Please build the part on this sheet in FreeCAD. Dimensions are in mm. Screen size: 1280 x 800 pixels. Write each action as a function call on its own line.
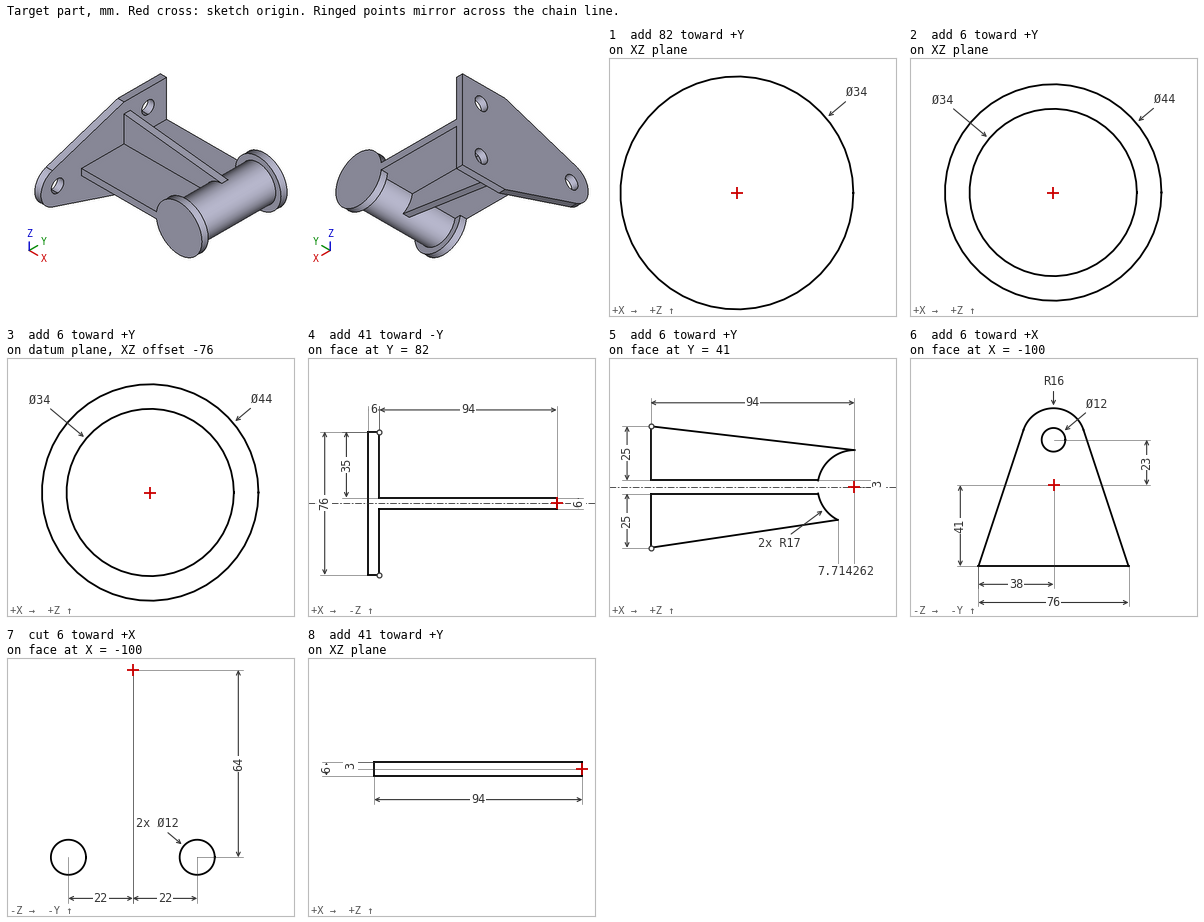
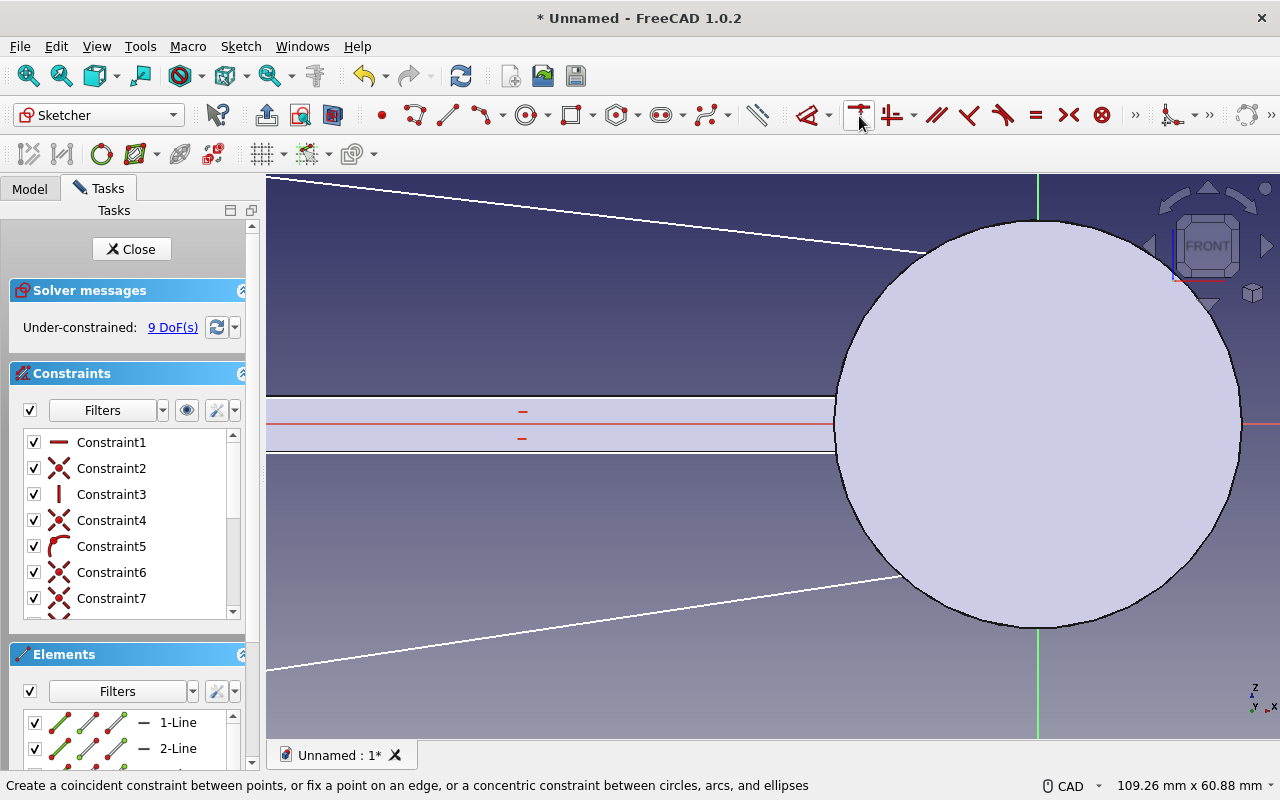
click(973, 280)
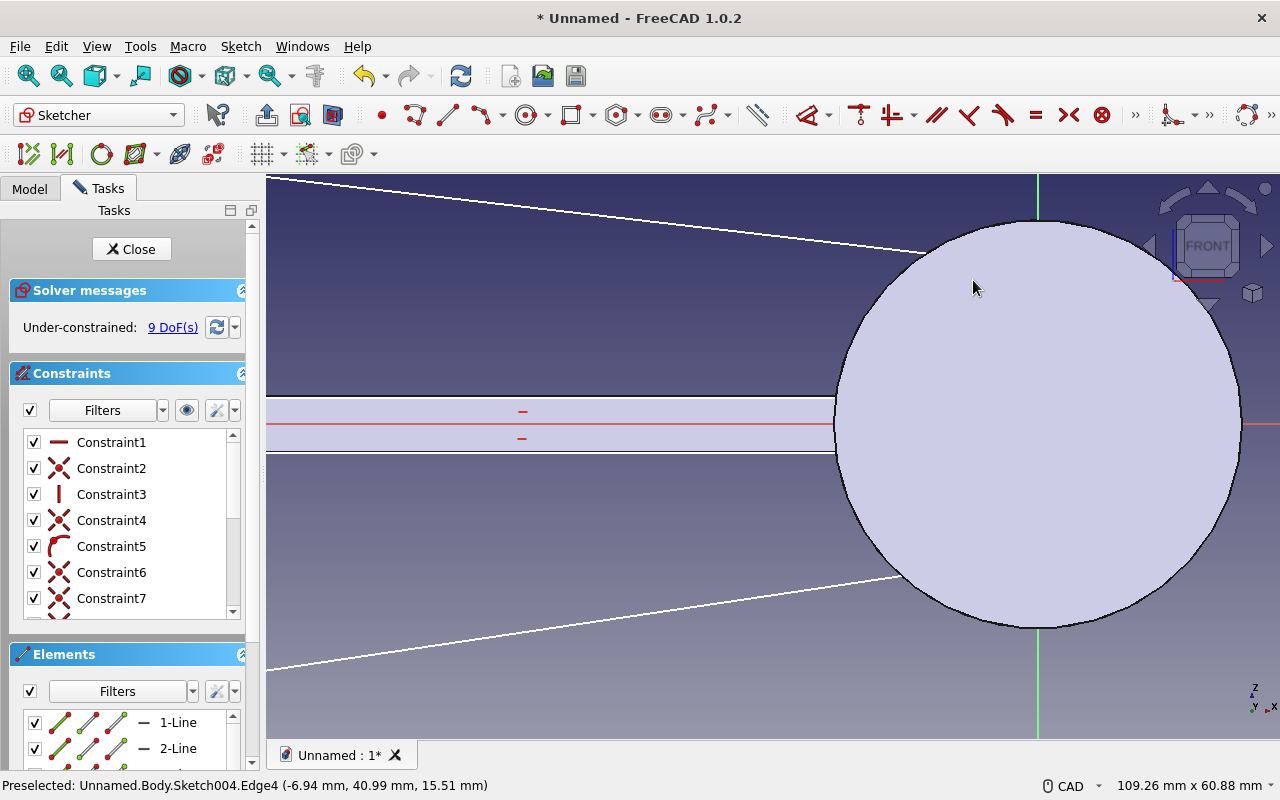
click(895, 495)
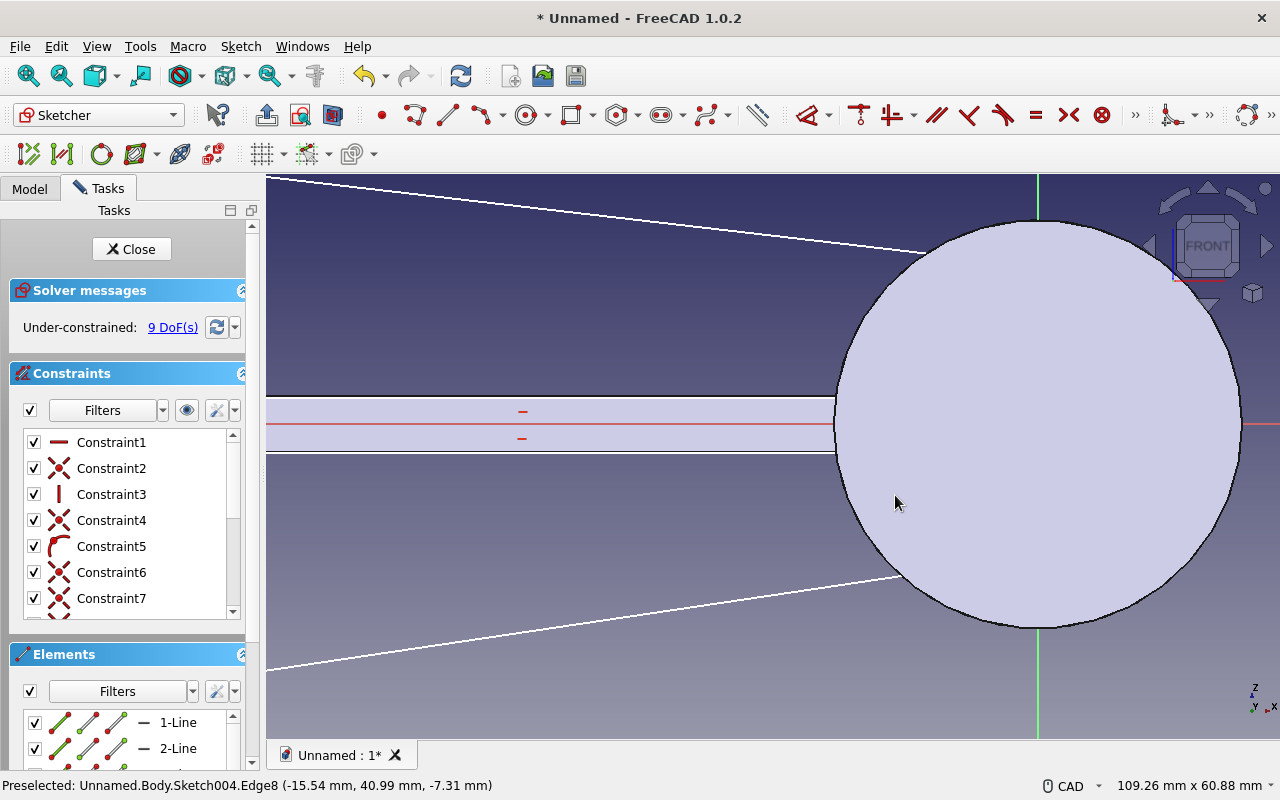
click(1036, 116)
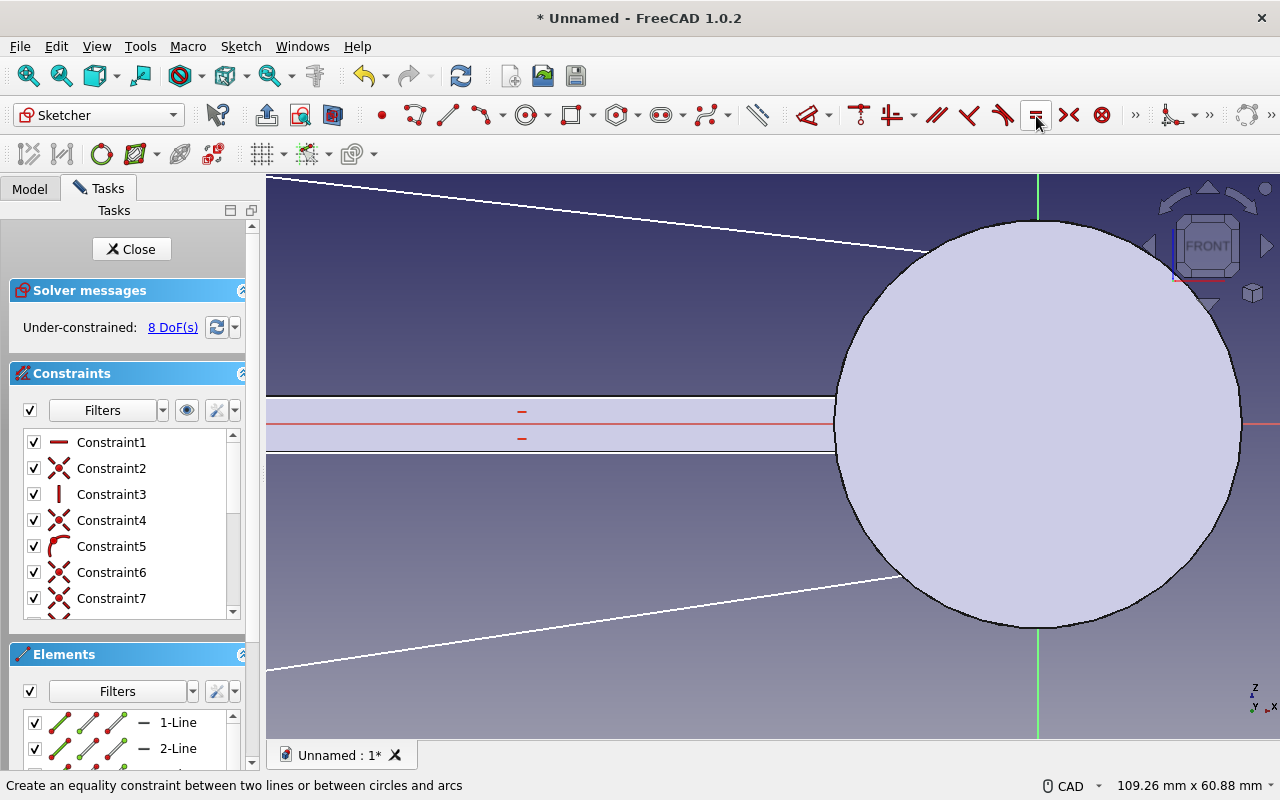
scroll(913, 522, down, 2)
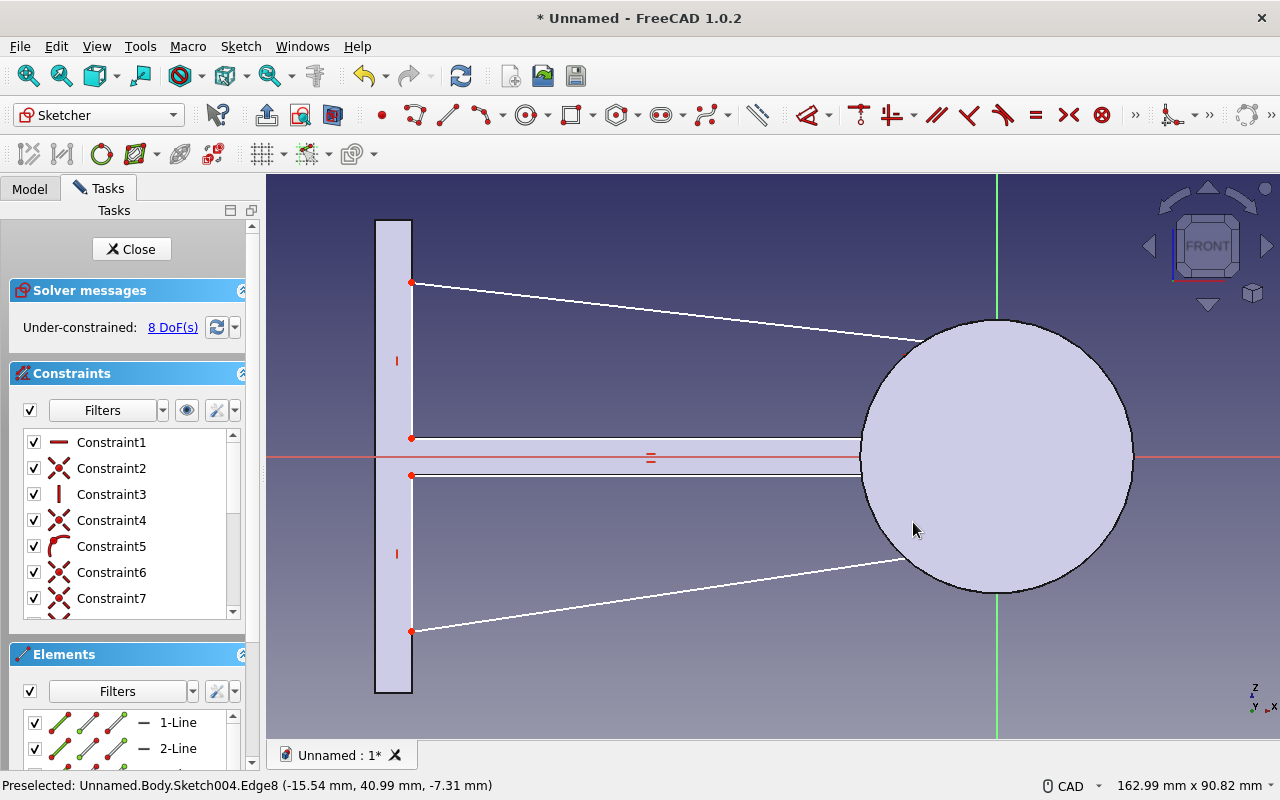
click(412, 283)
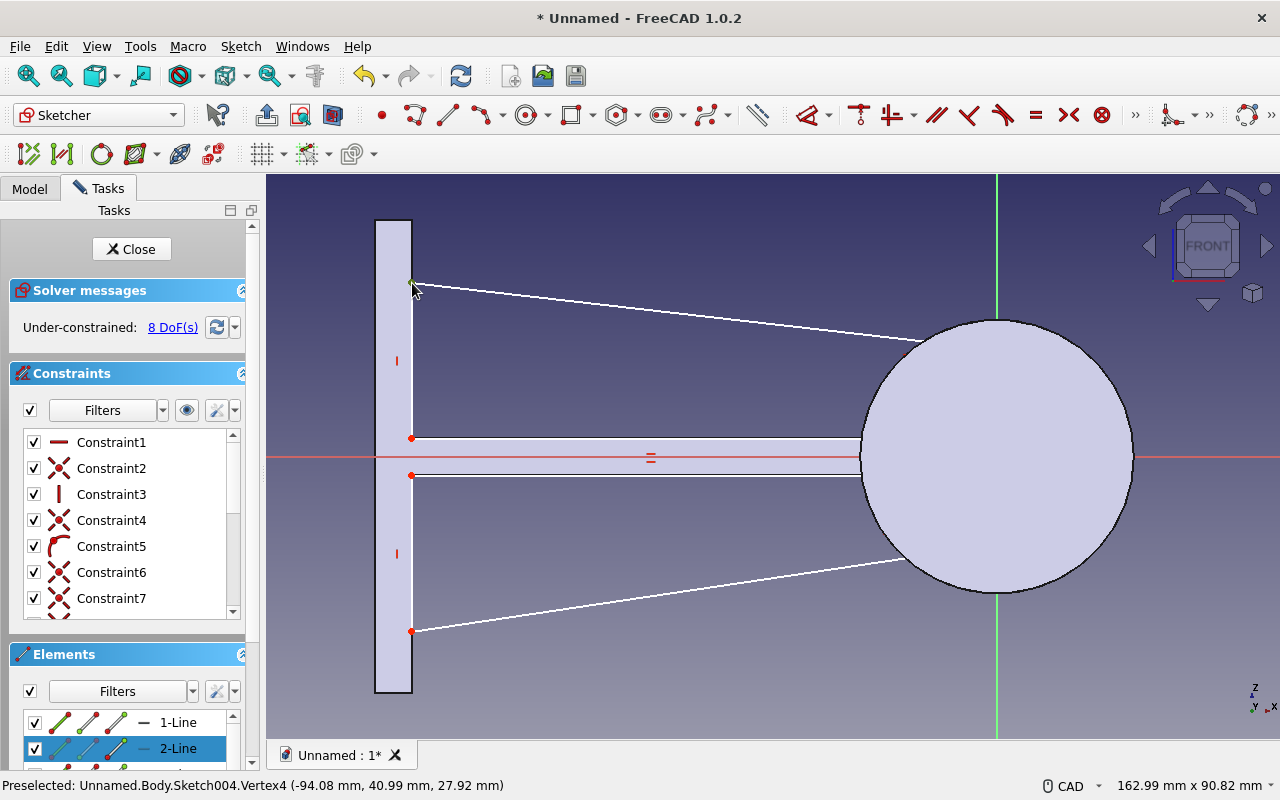
click(412, 632)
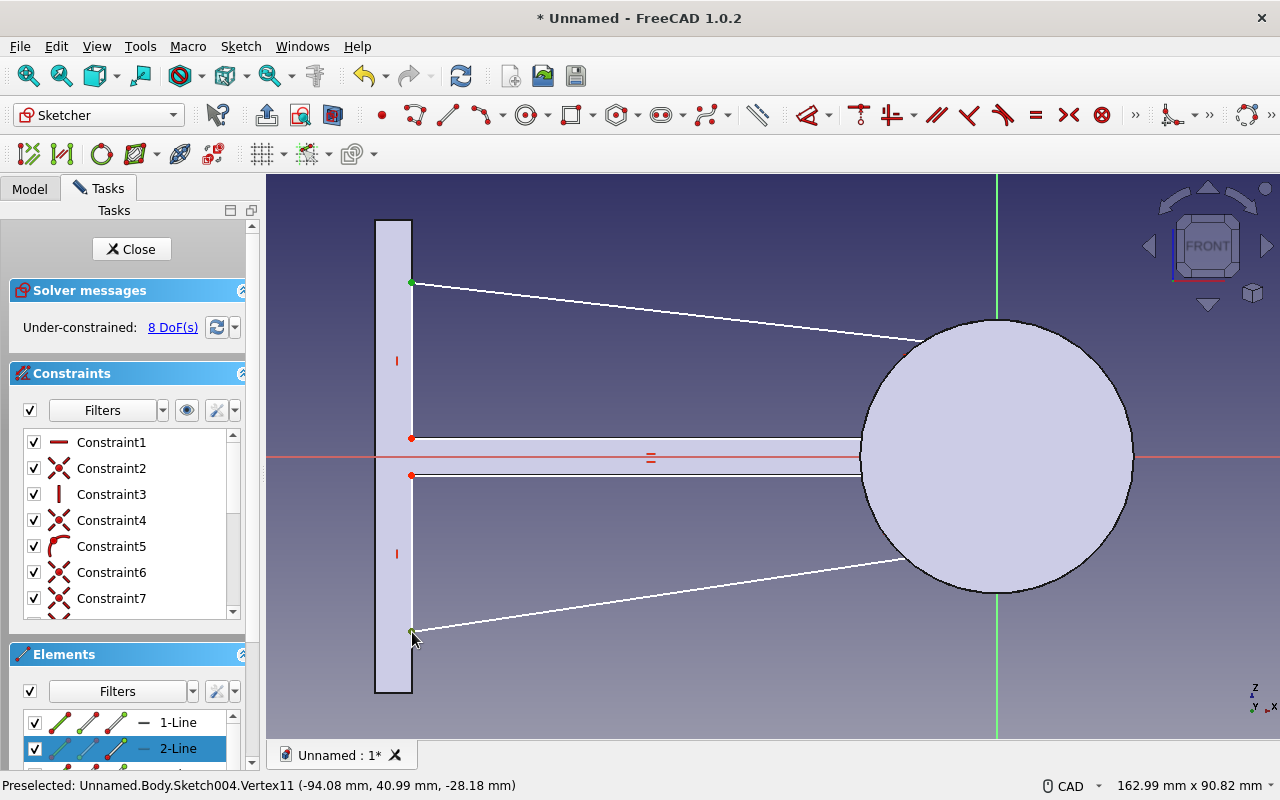
click(353, 457)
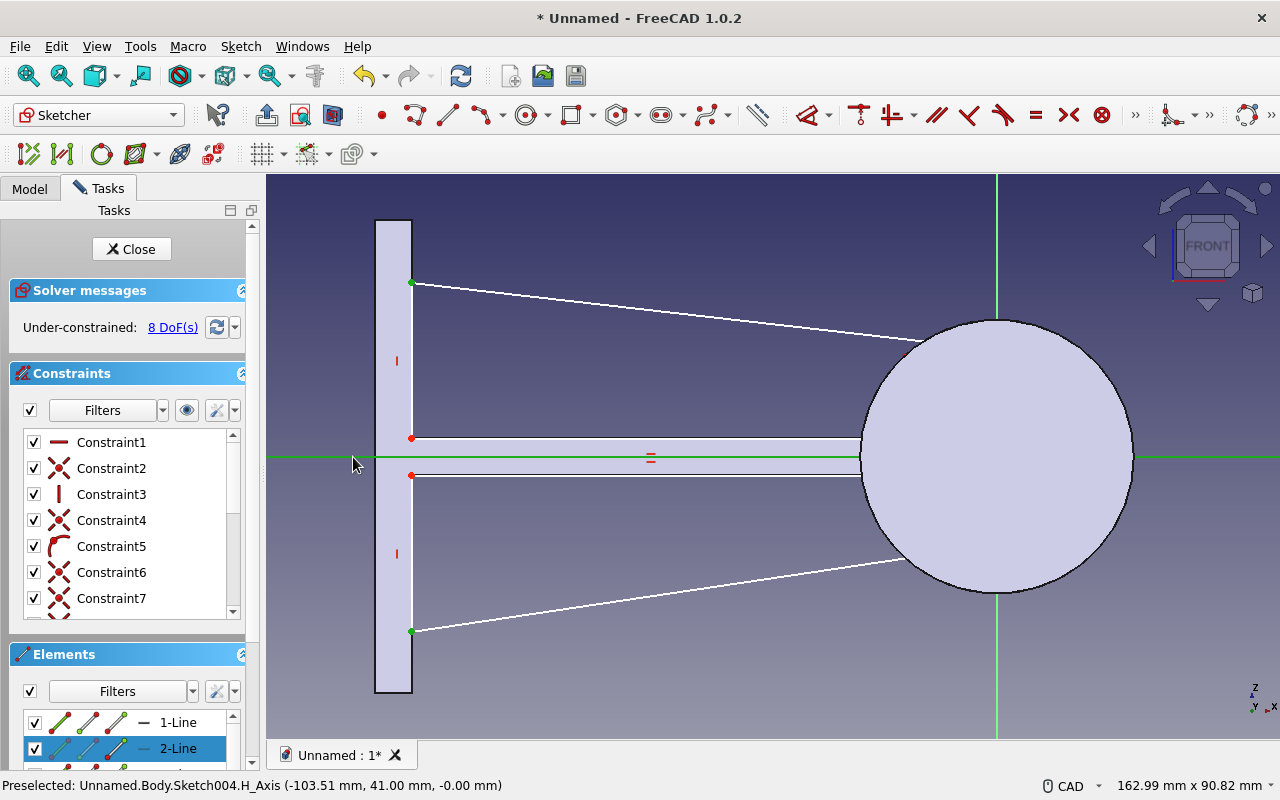
click(1069, 116)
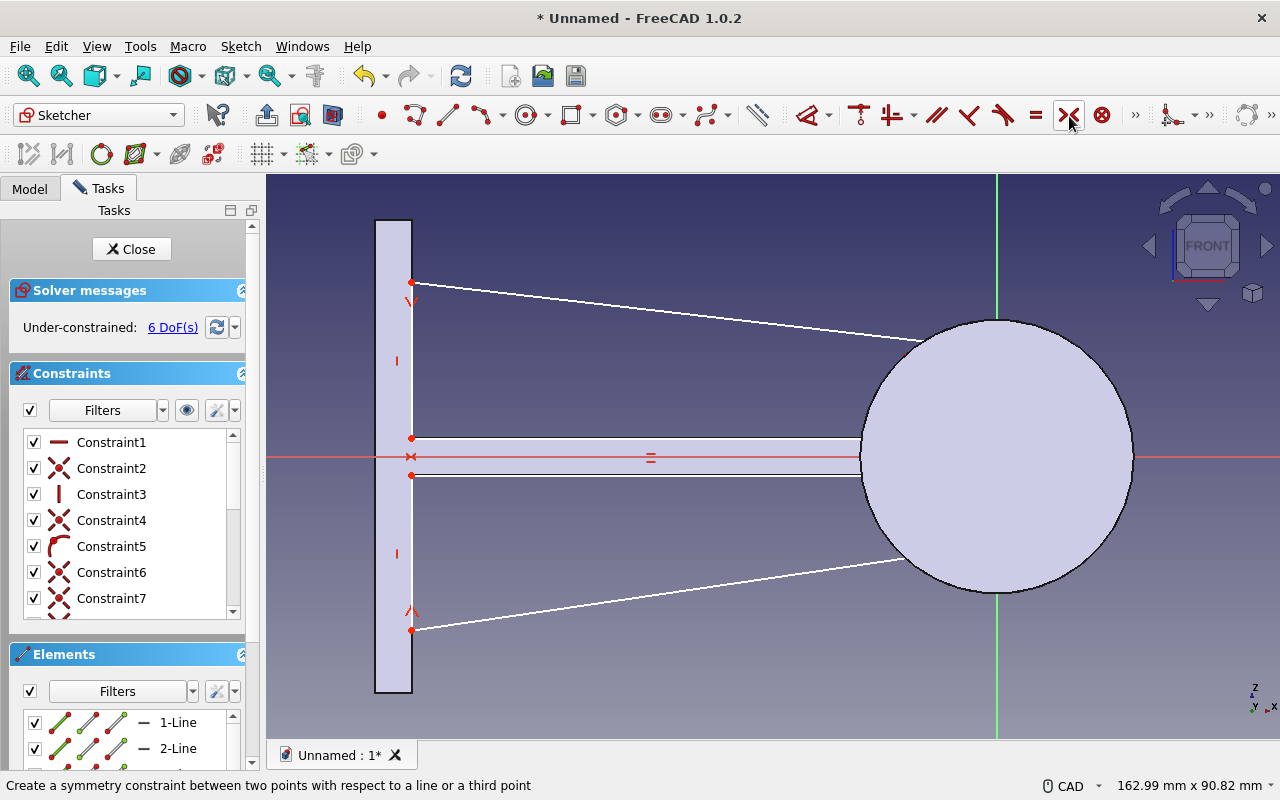
click(806, 116)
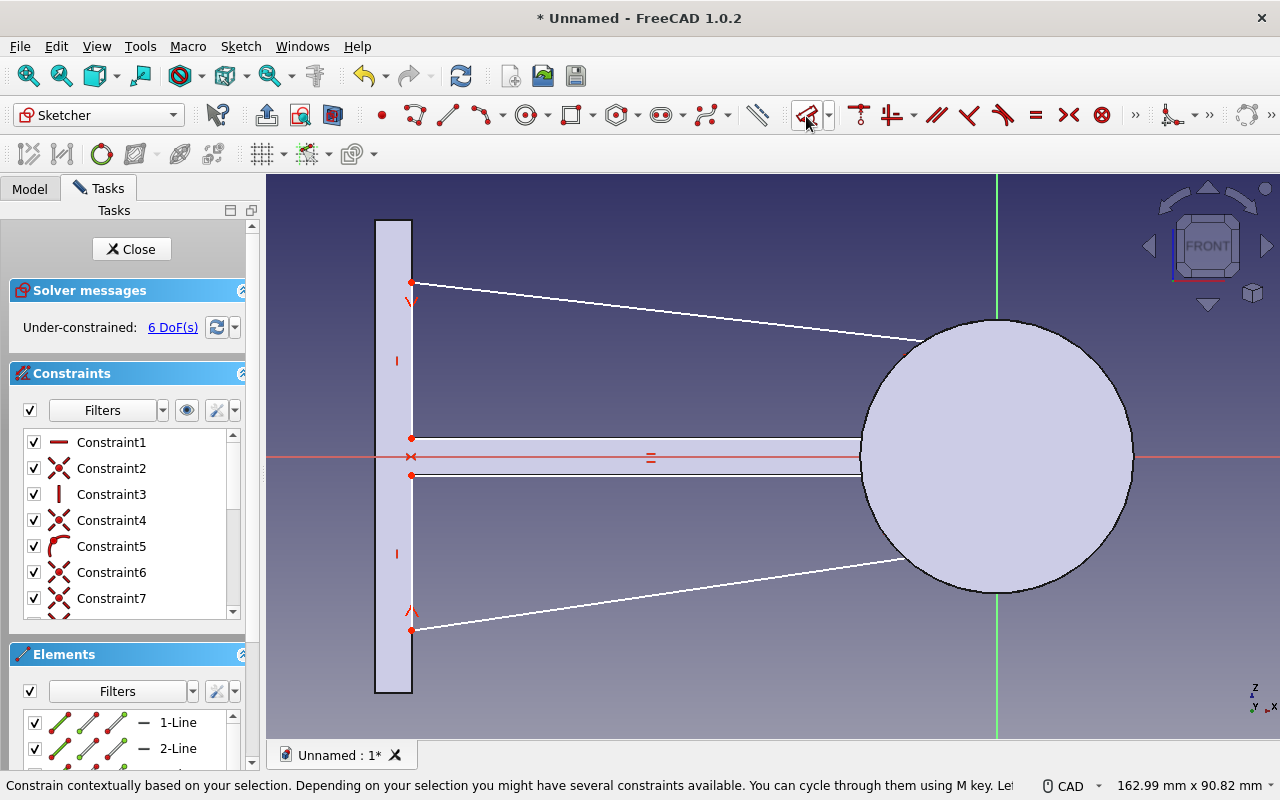
click(953, 359)
click(940, 330)